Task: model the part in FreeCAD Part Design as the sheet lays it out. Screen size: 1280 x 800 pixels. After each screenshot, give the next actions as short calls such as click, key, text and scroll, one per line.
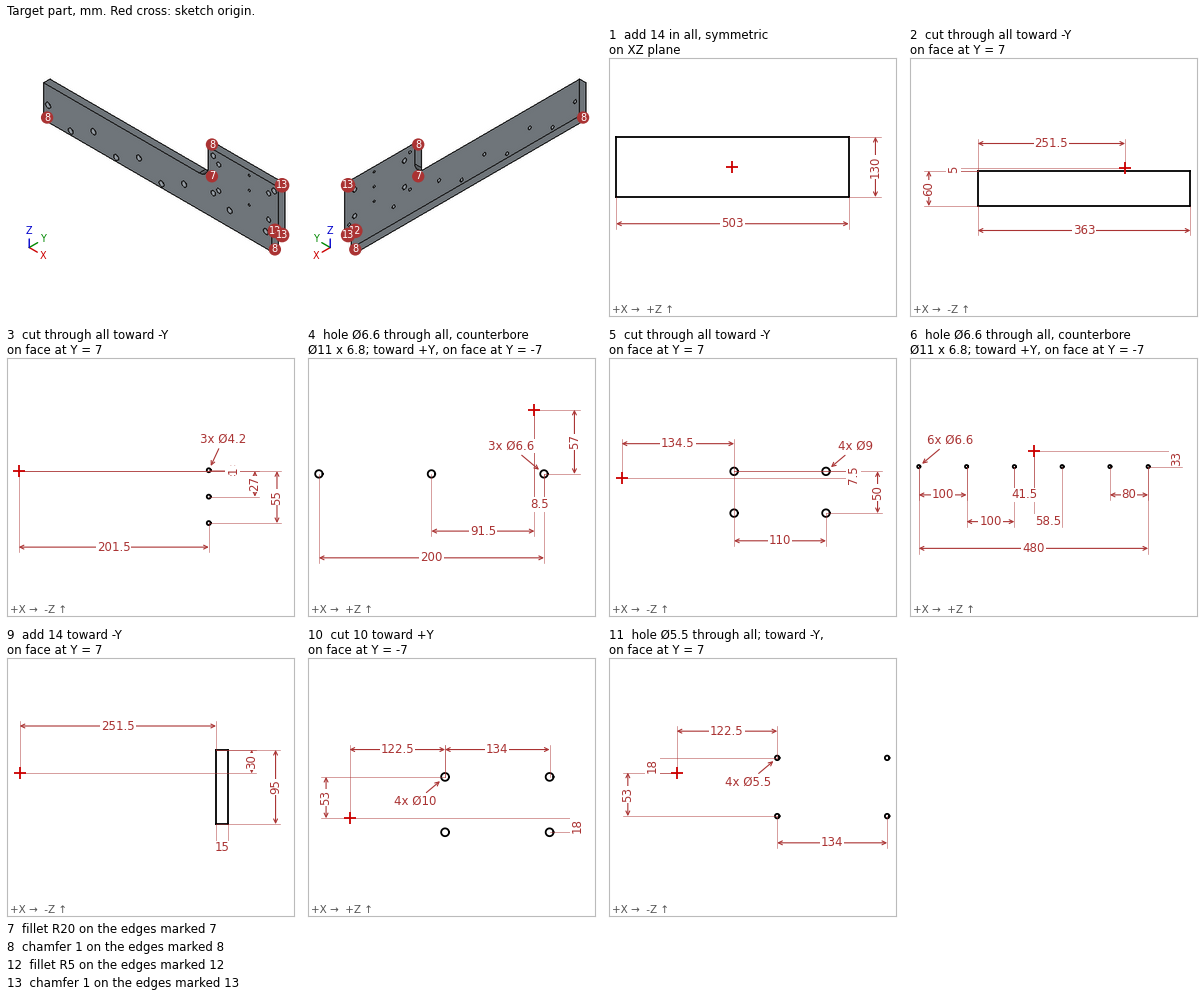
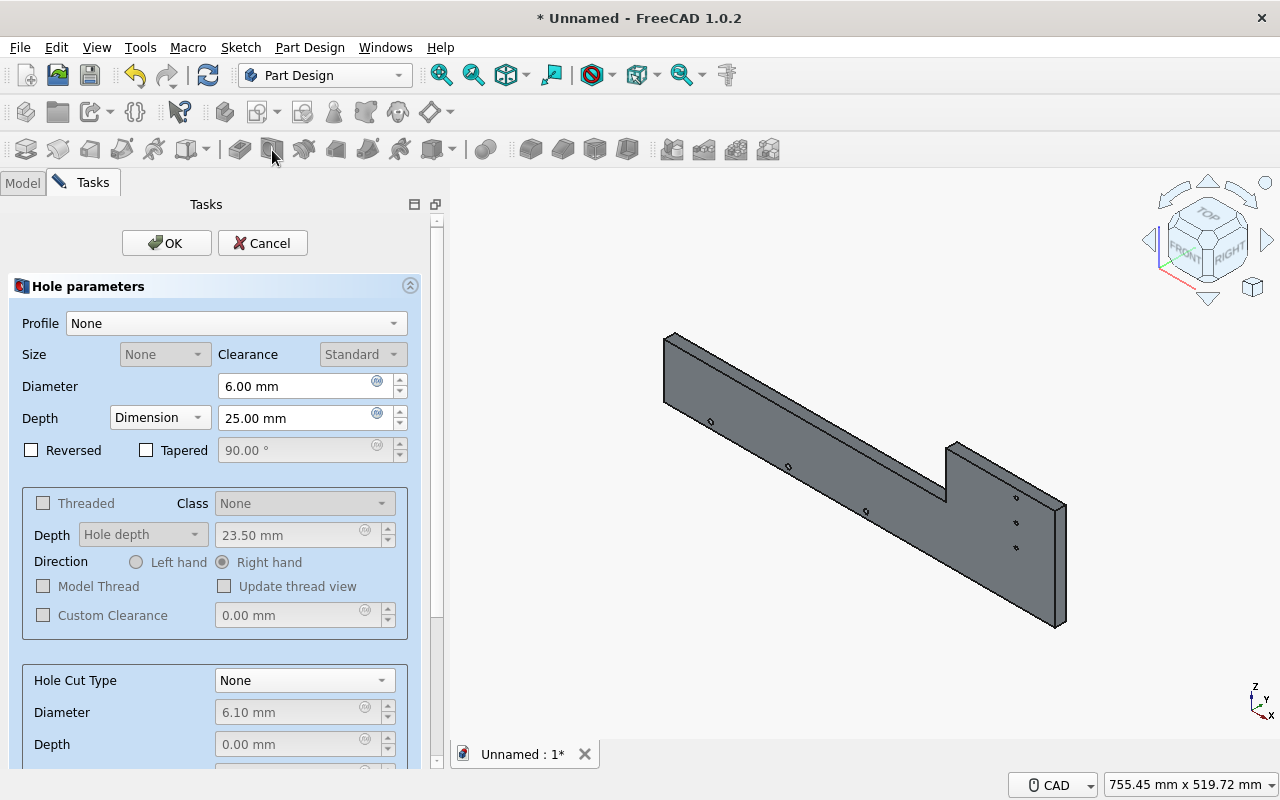
triple_click(305, 386)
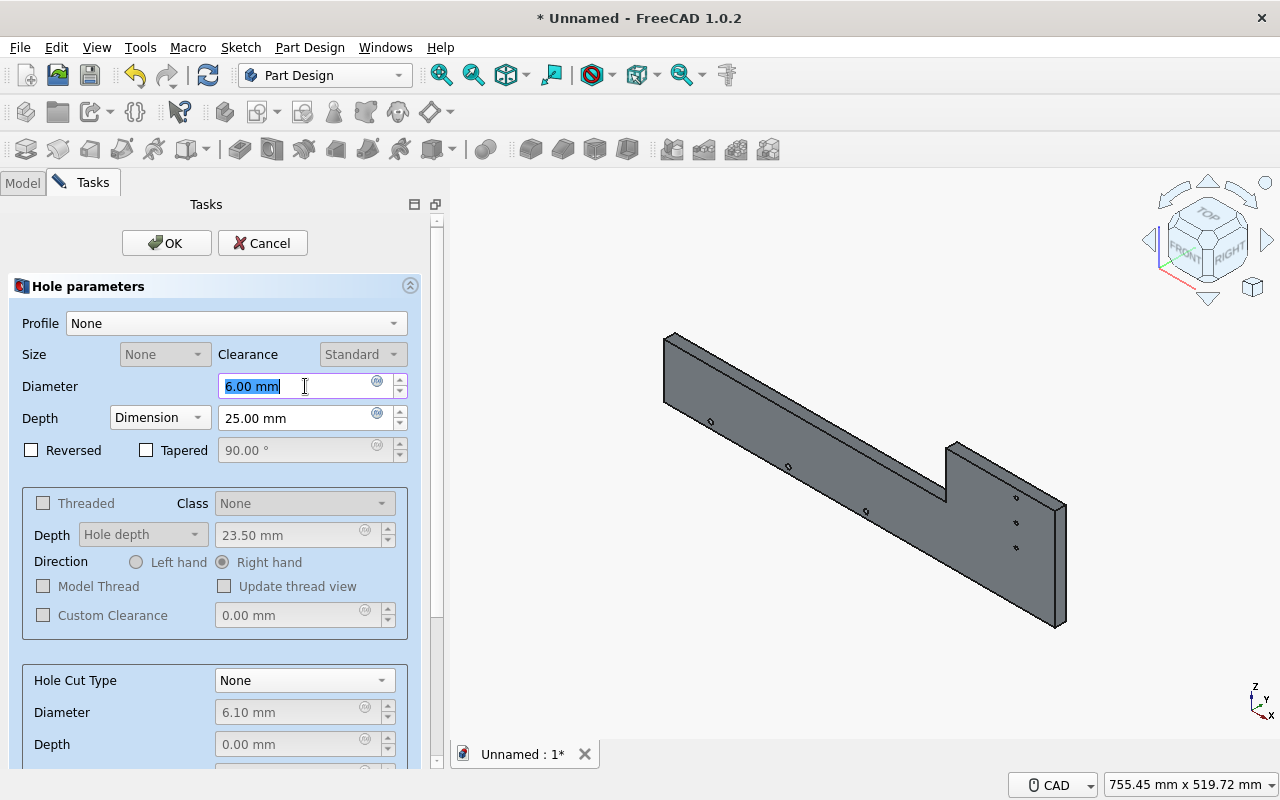
text(6.6)
key(Tab)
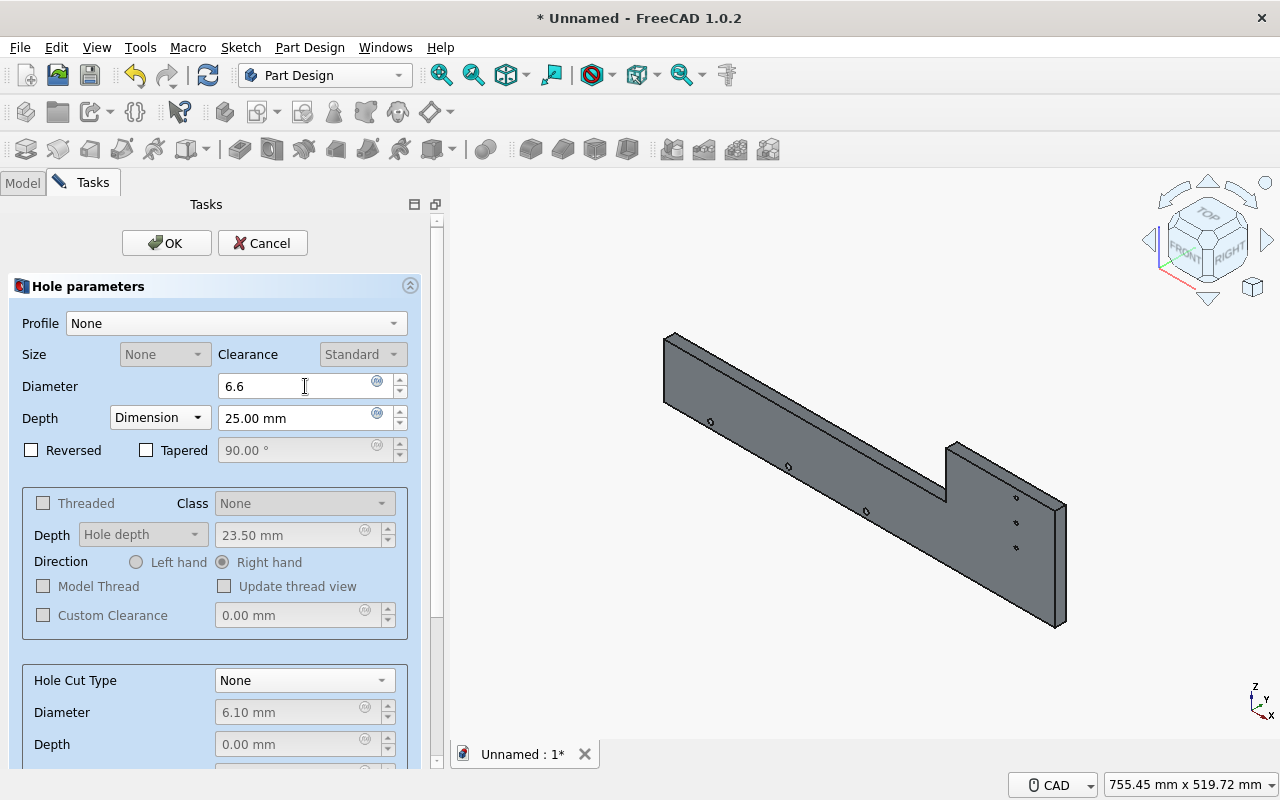
click(161, 418)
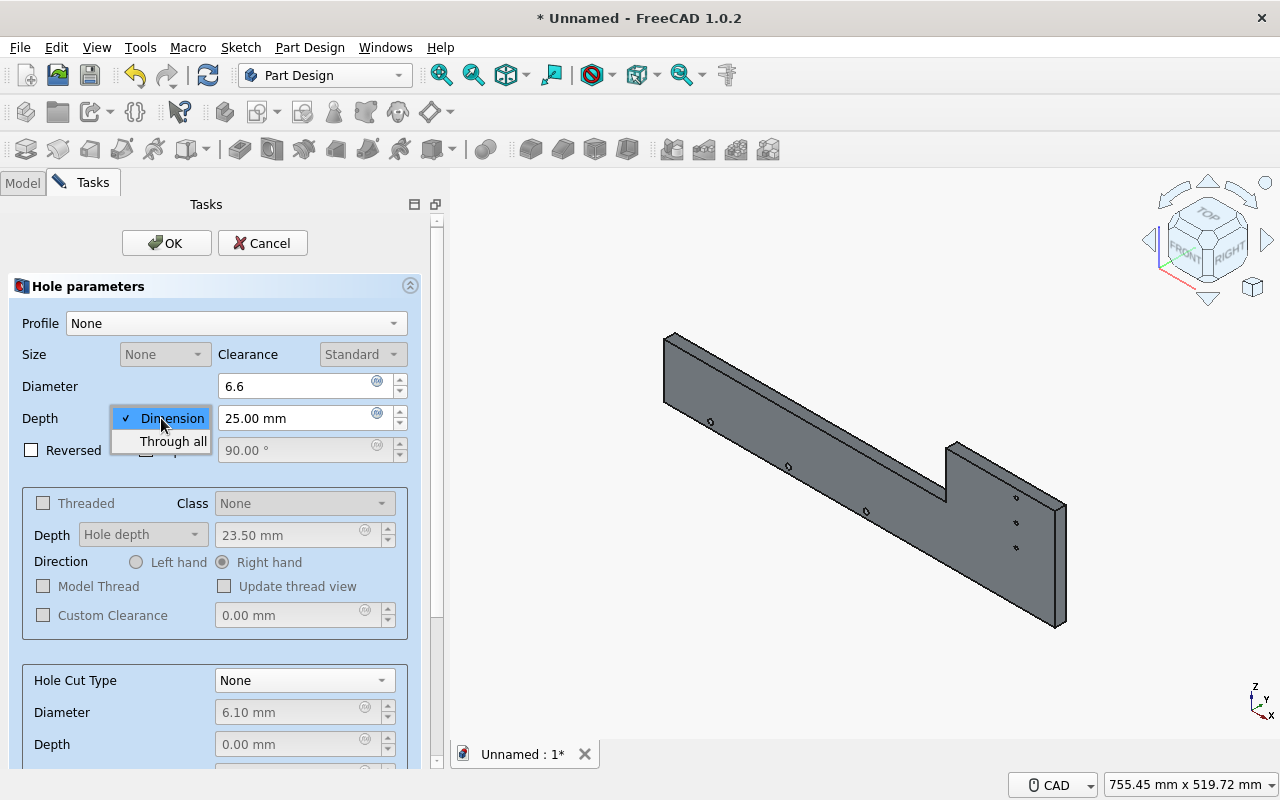
click(160, 442)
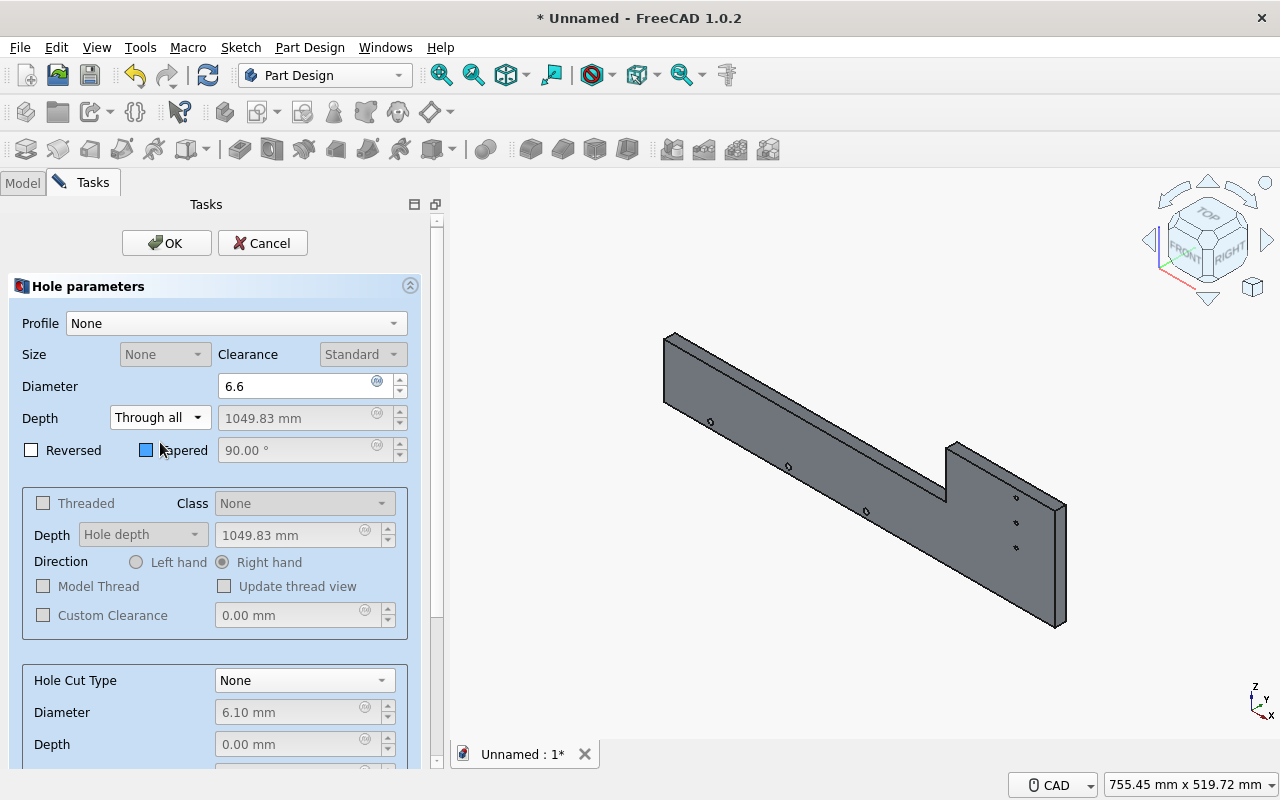
click(306, 680)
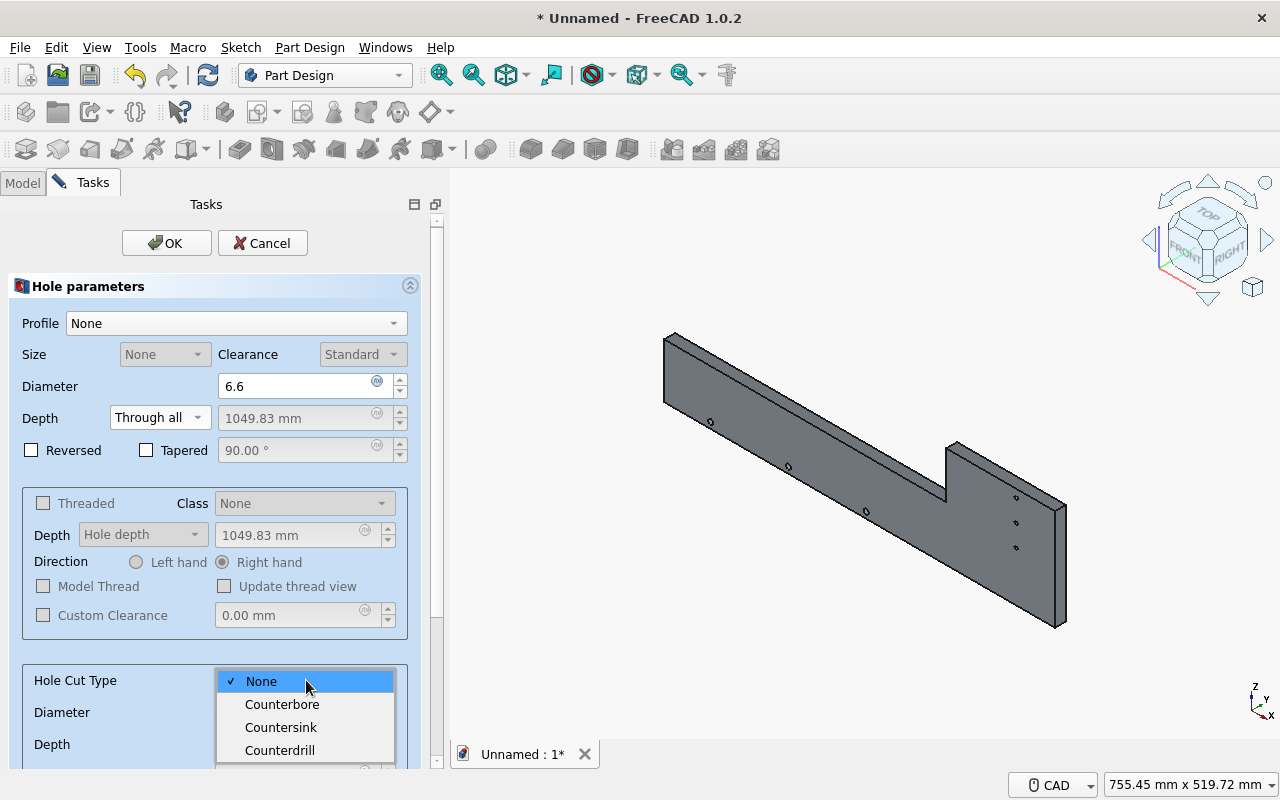
click(304, 704)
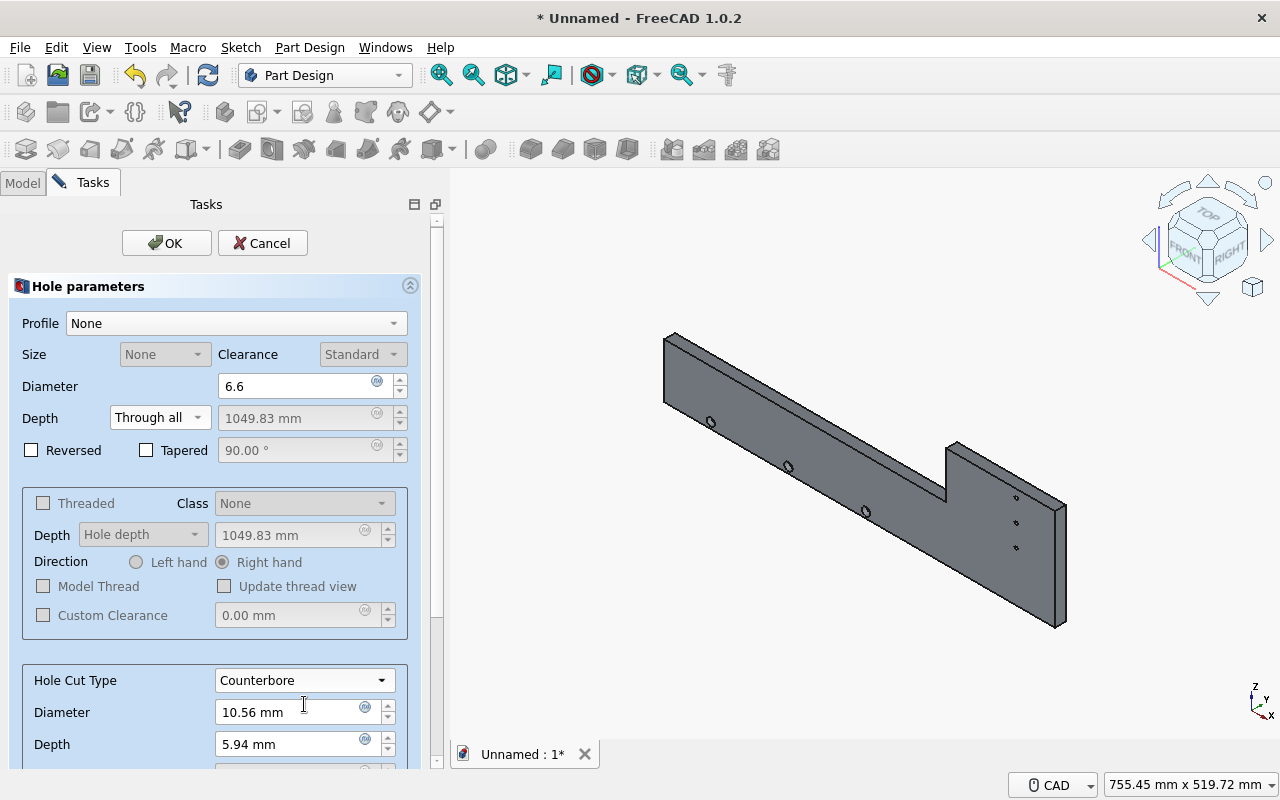
triple_click(298, 712)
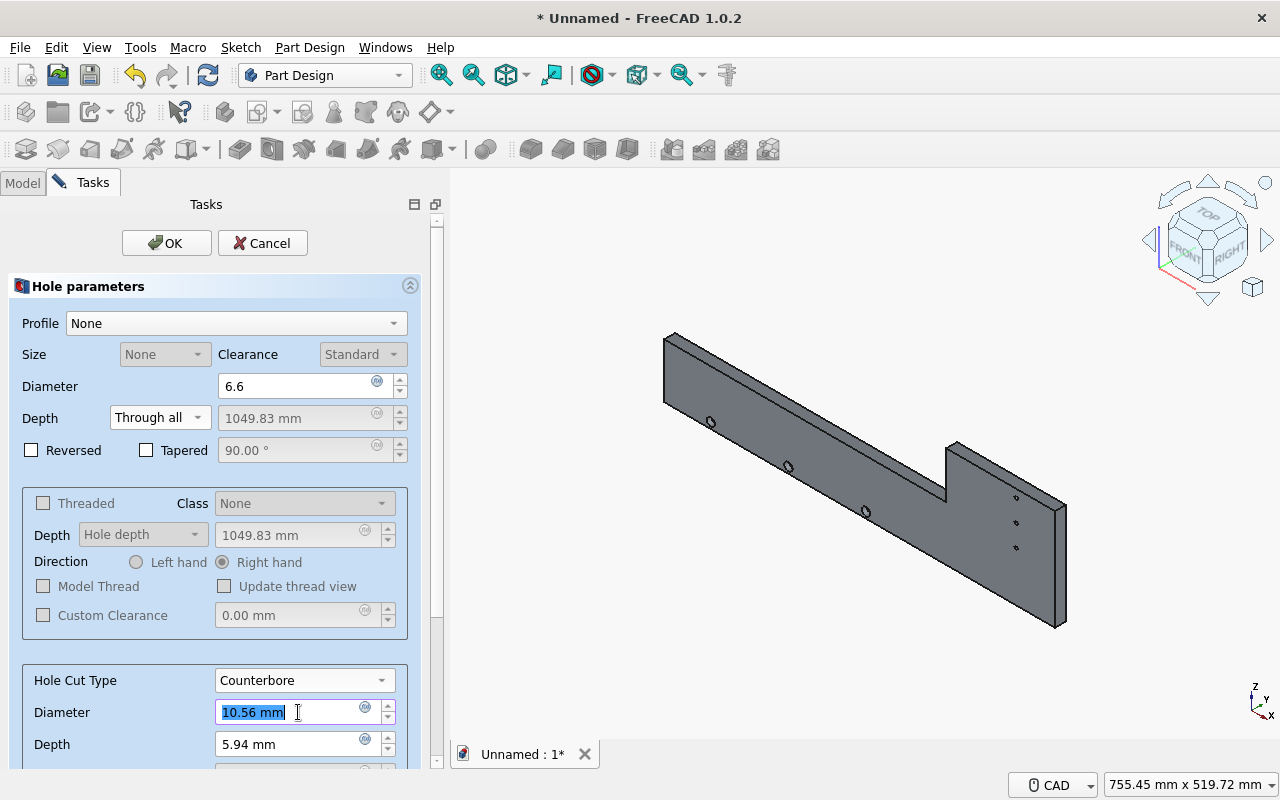
text(11)
key(Tab)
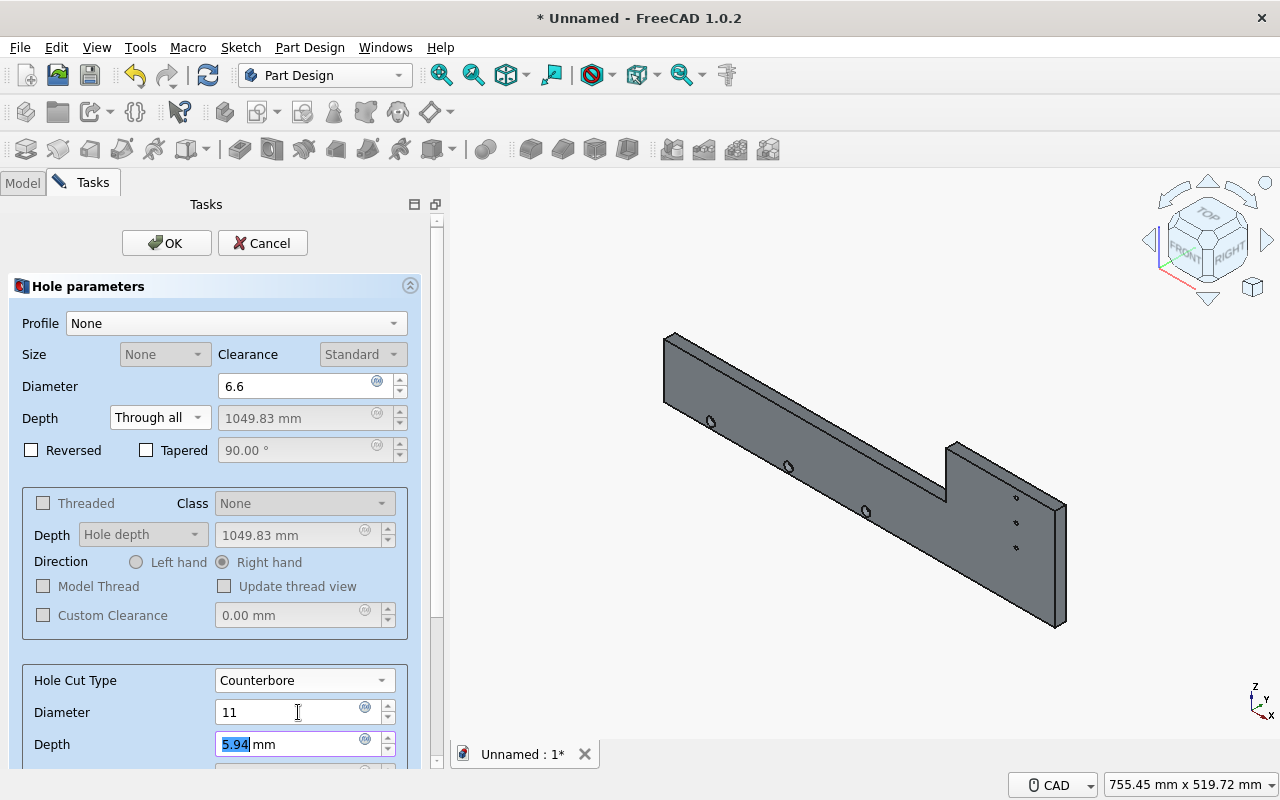
text(6.8)
key(Tab)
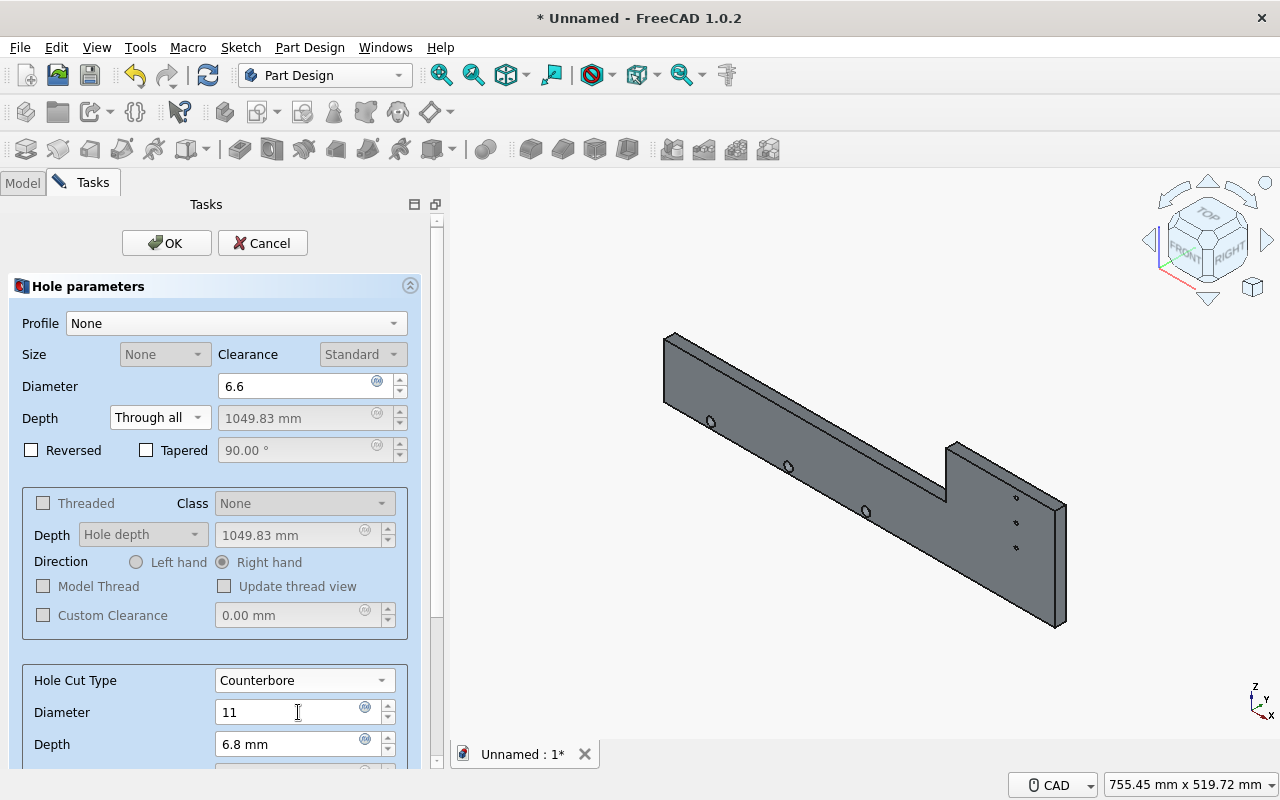
click(167, 243)